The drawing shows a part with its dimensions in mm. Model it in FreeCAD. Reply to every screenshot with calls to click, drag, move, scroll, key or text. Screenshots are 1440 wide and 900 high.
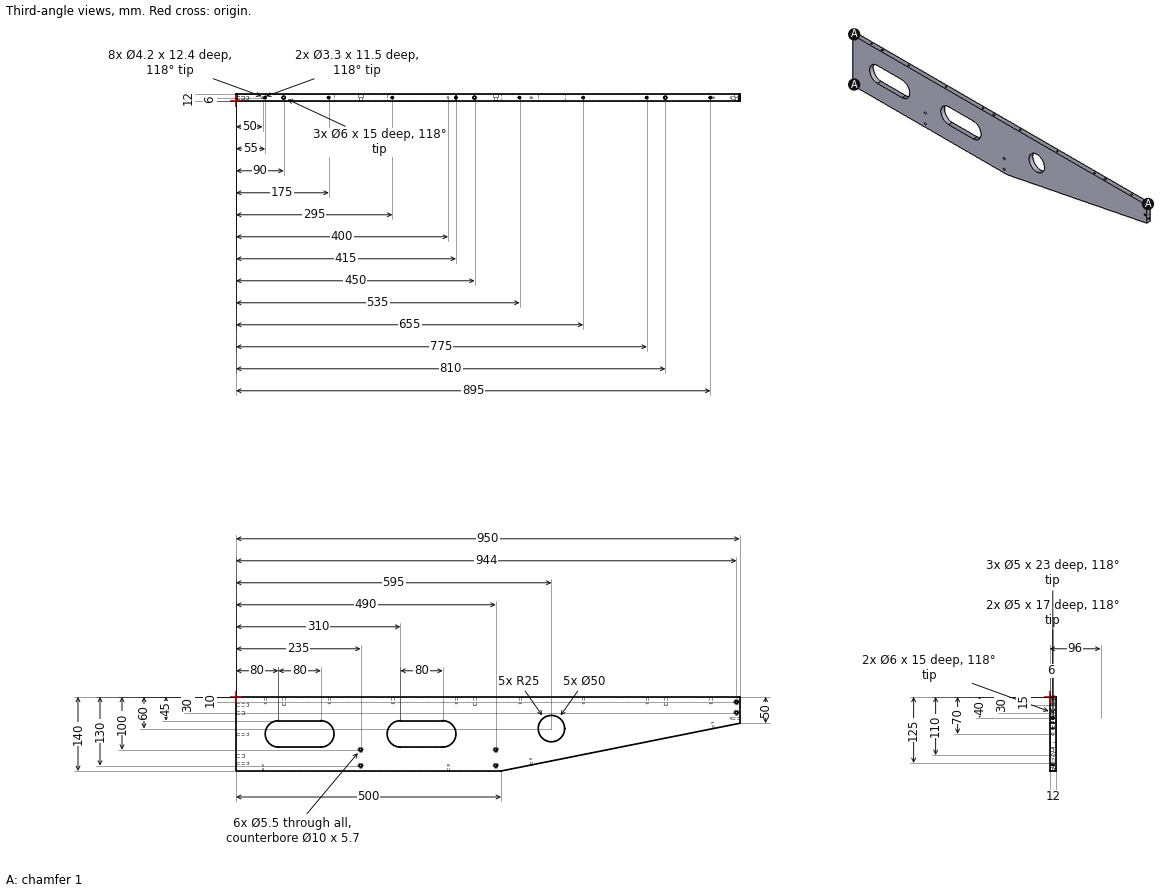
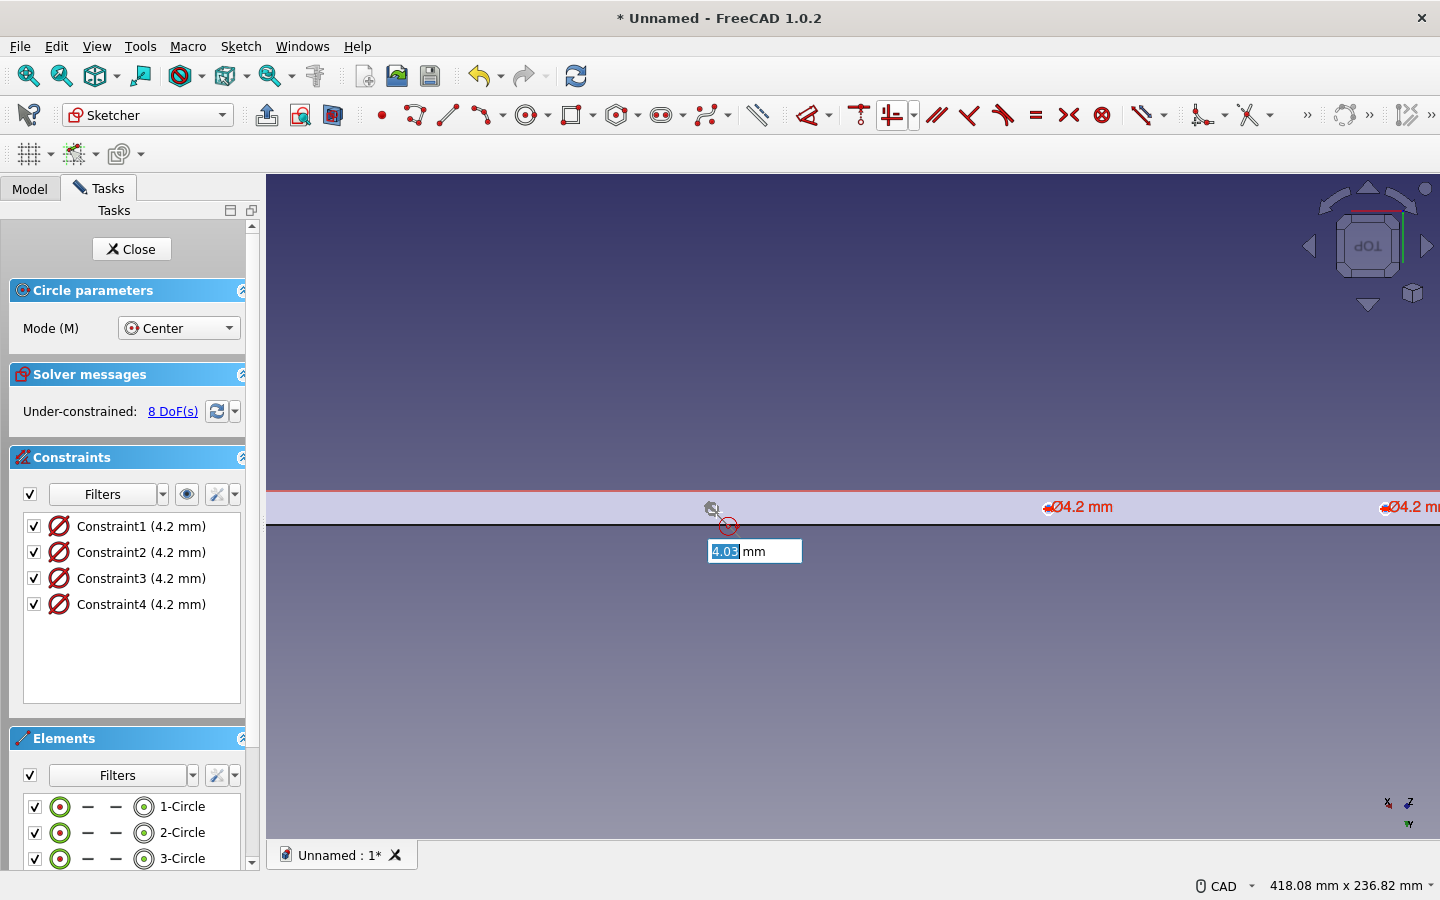
text(4.2)
key(Return)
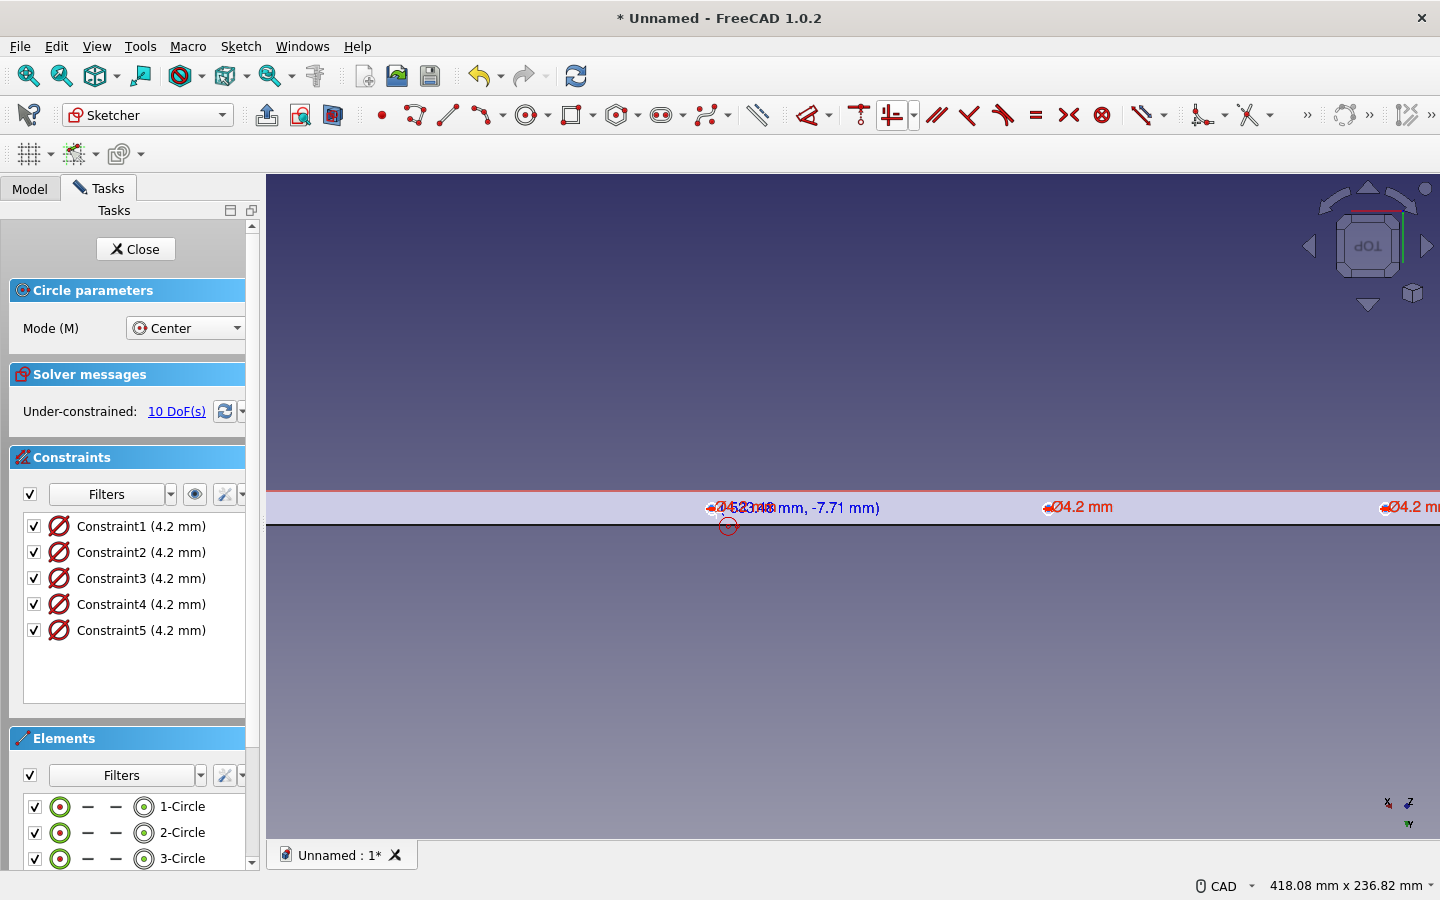
scroll(375, 508, up, 7)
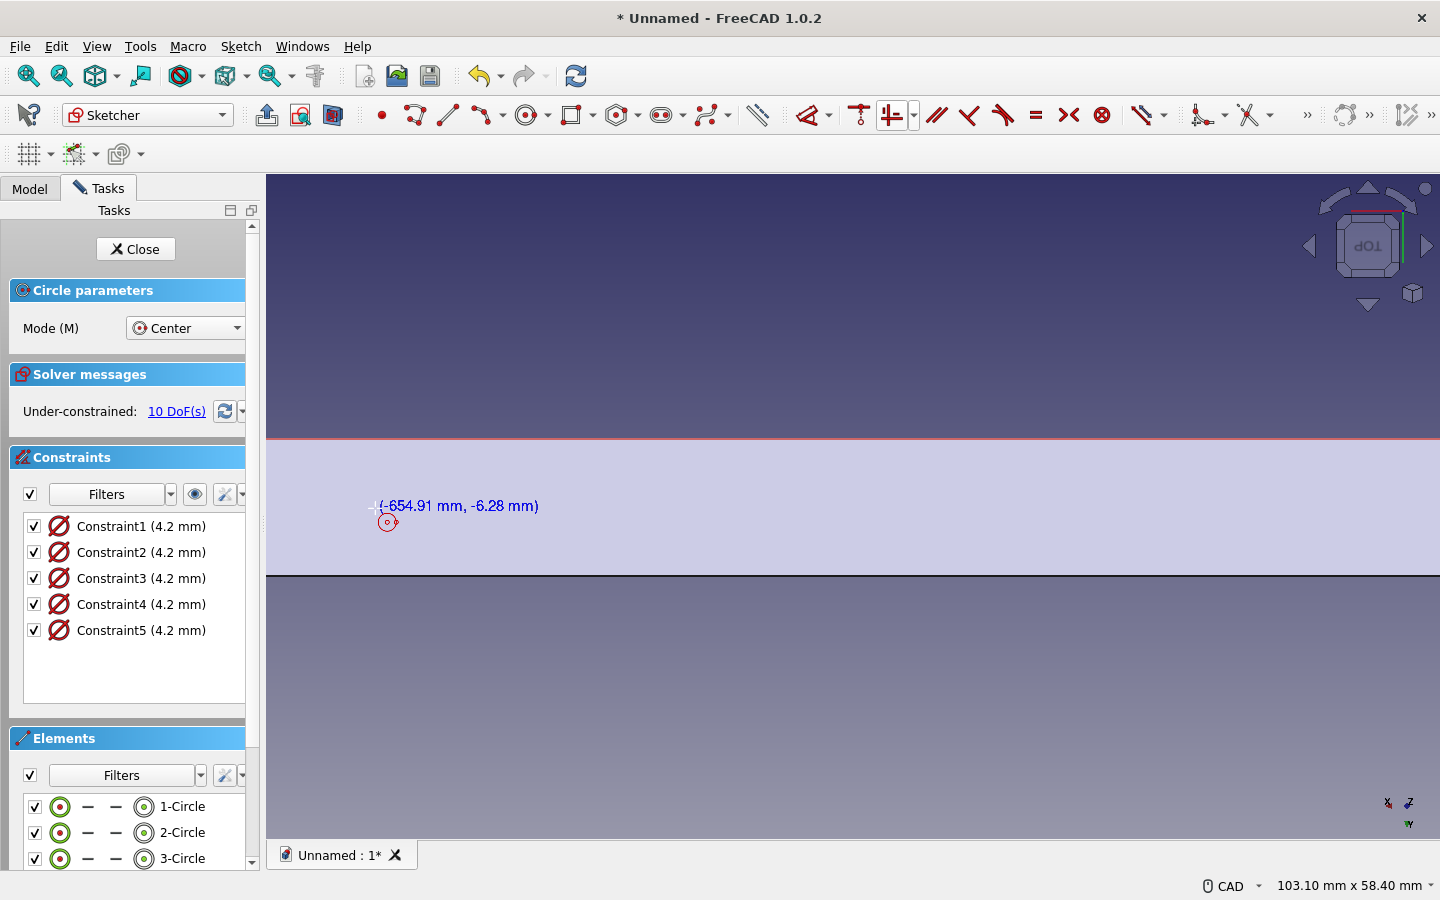
scroll(629, 508, down, 13)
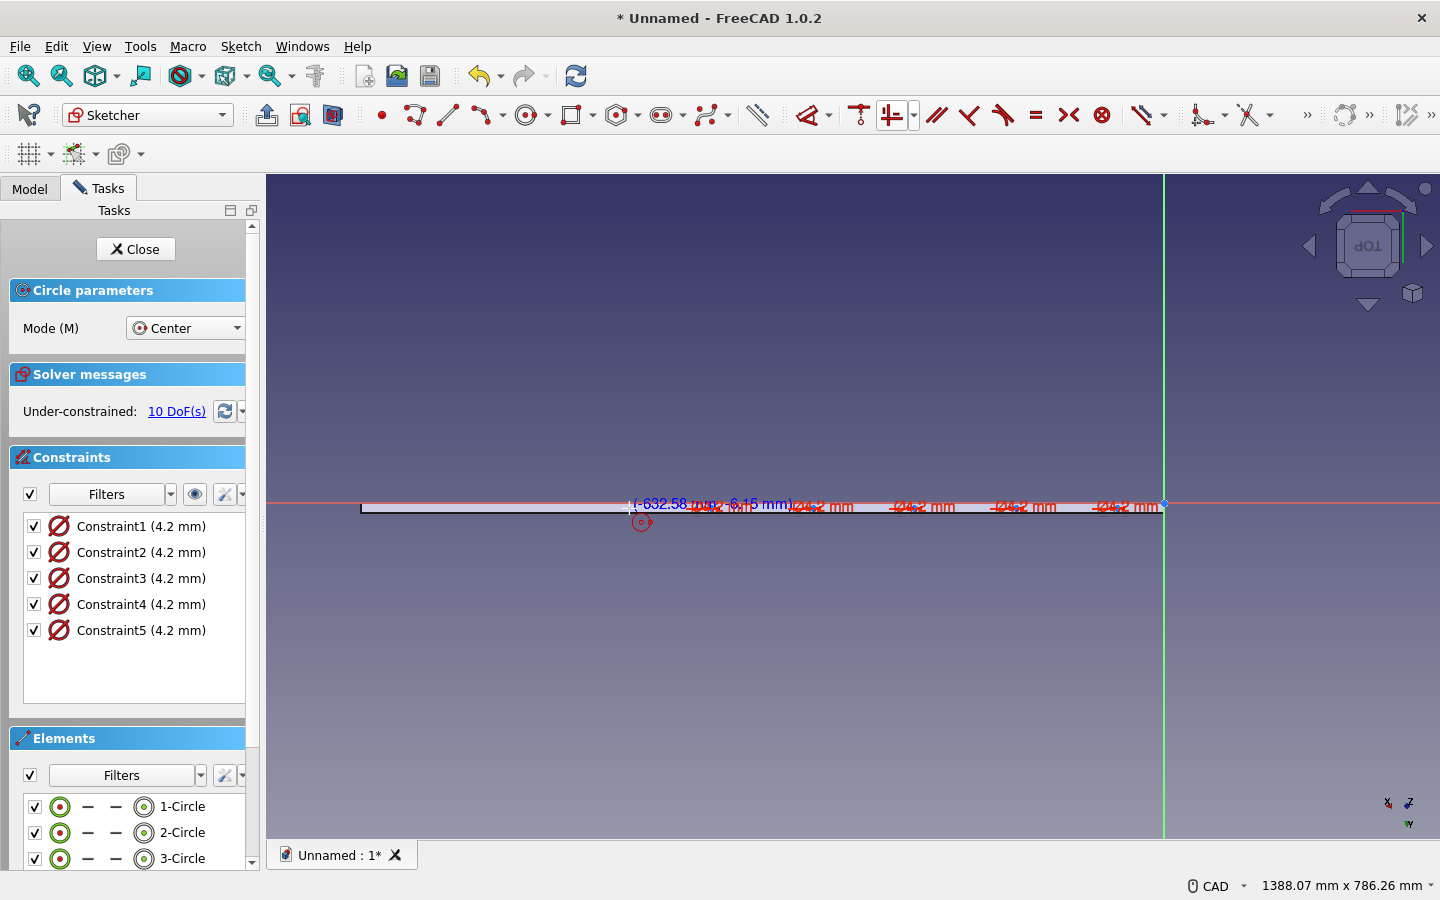
scroll(610, 508, up, 6)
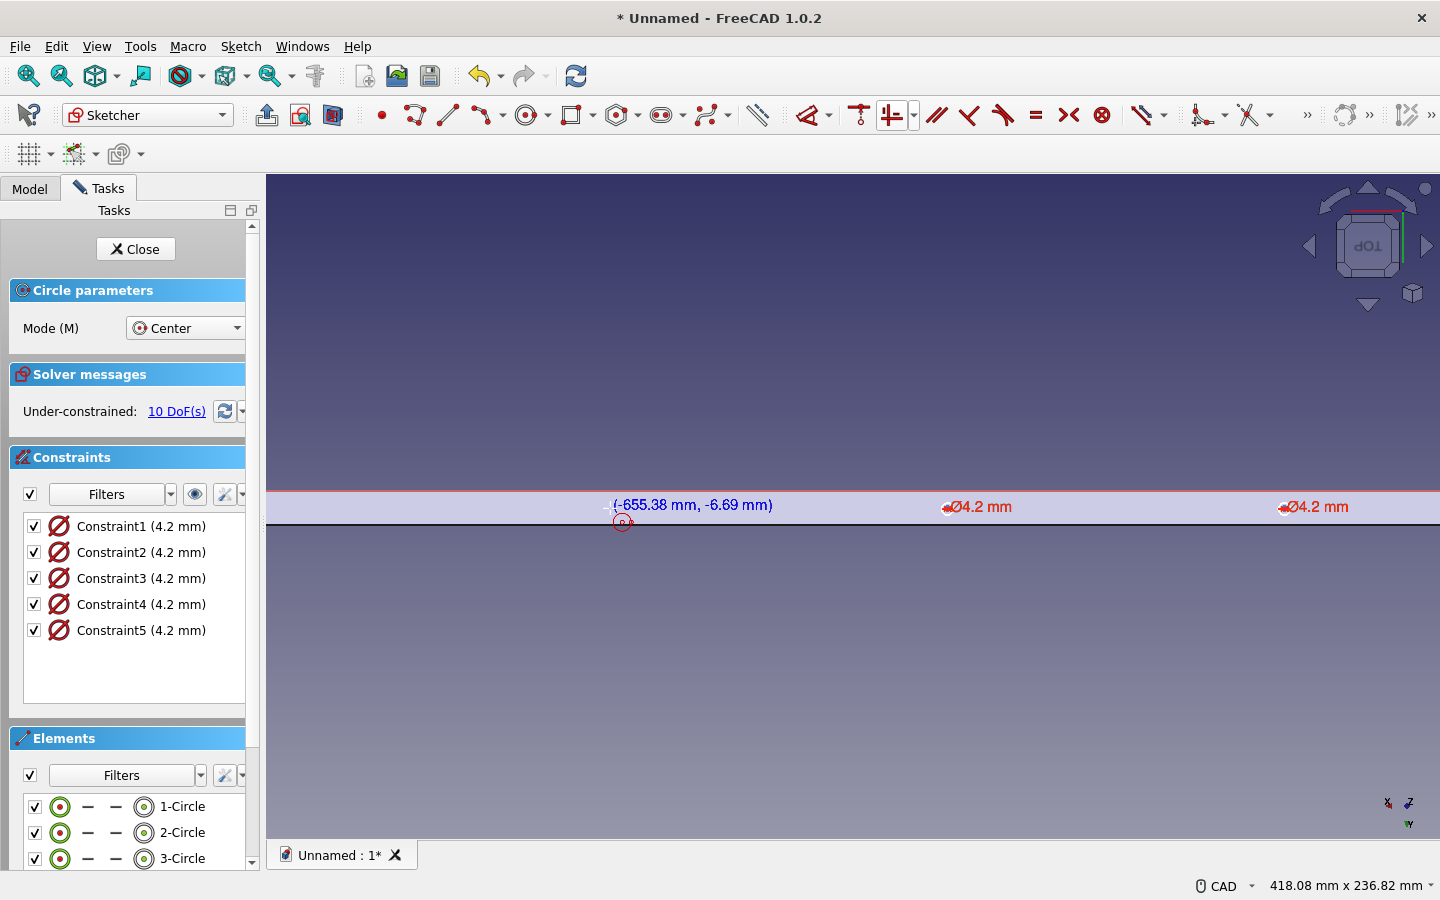
click(610, 508)
move(615, 512)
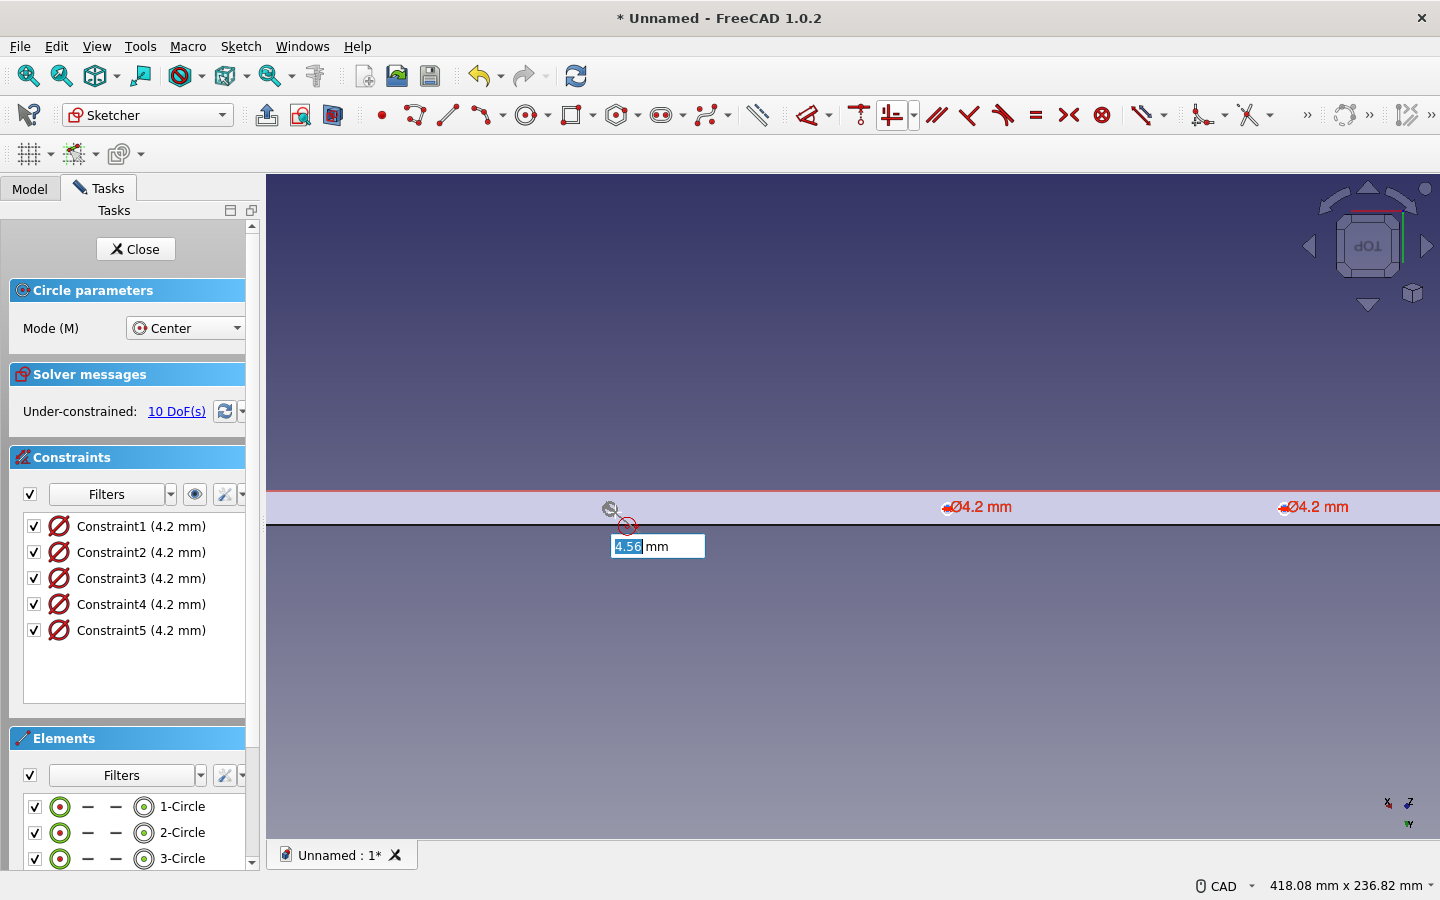
text(4.2)
key(Return)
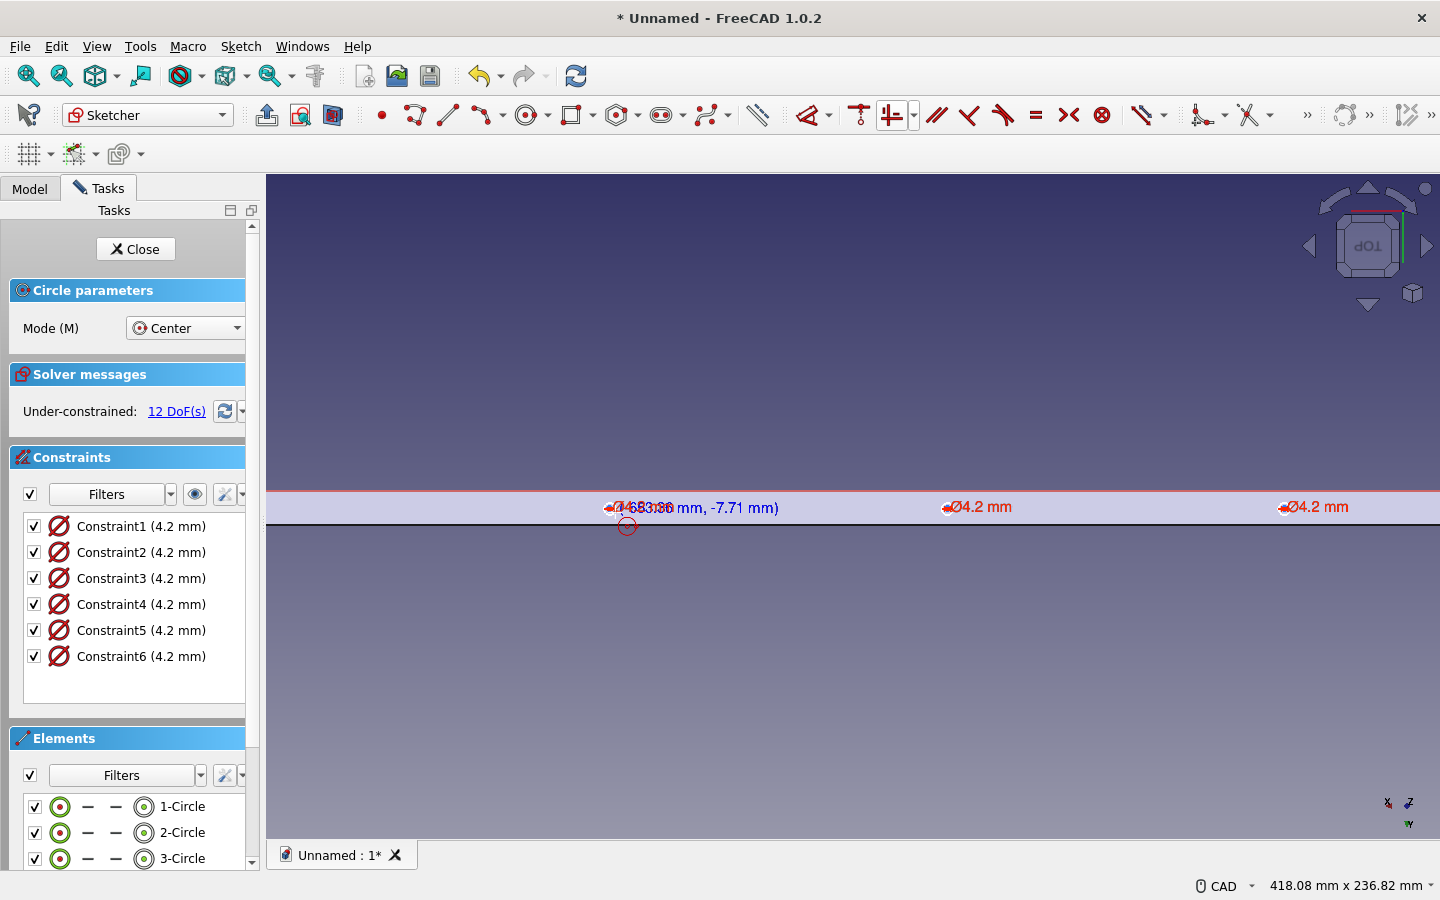
scroll(610, 508, down, 6)